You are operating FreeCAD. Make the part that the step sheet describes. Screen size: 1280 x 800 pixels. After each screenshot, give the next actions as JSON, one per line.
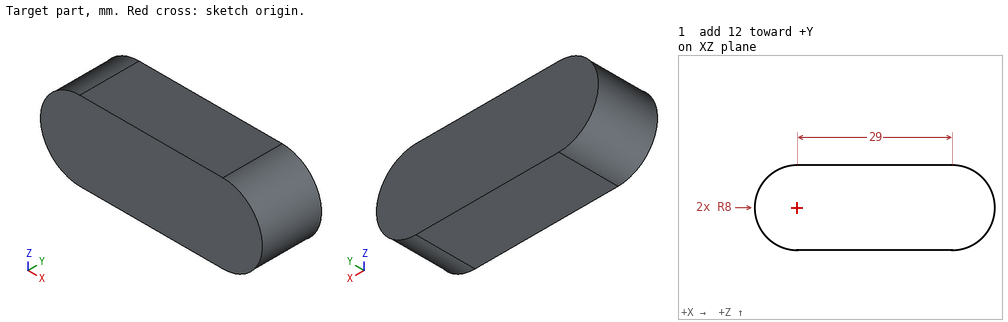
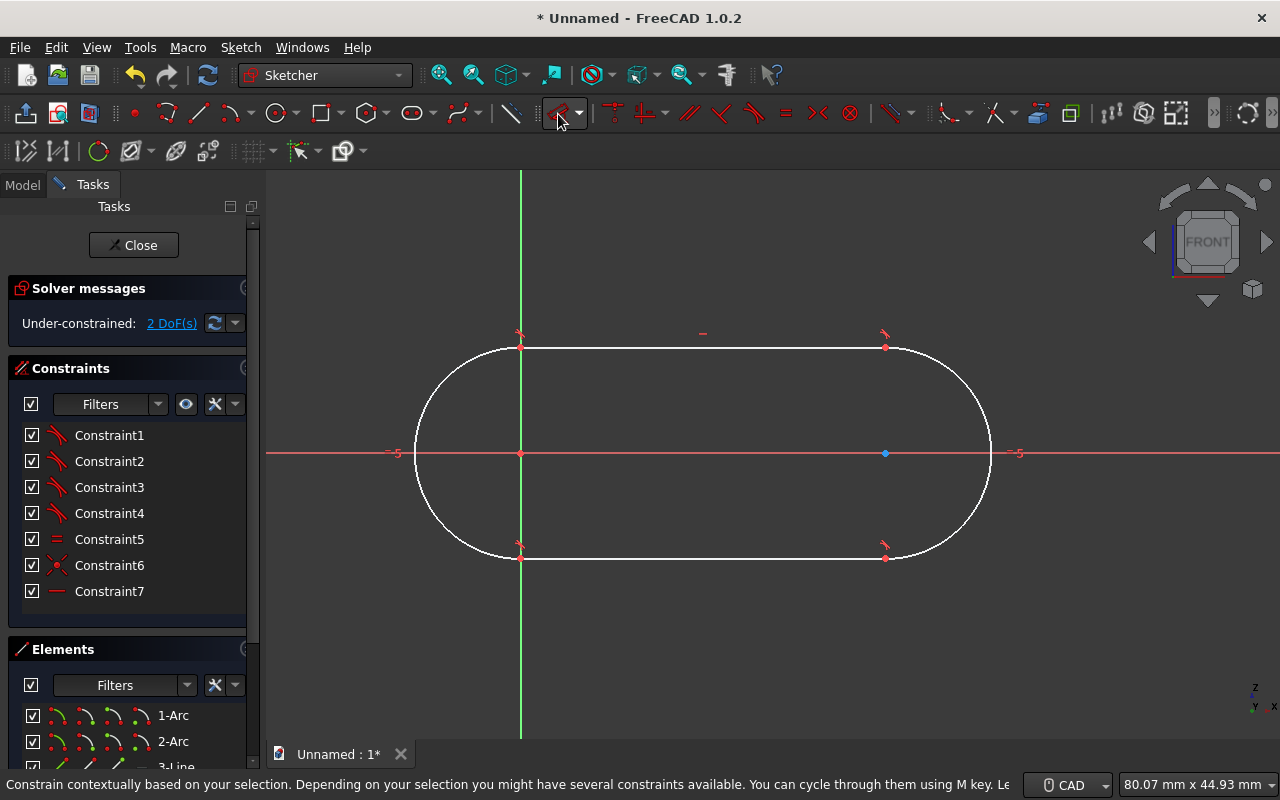
{"action": "left_click", "coordinate": [435, 391]}
{"action": "left_click", "coordinate": [409, 372]}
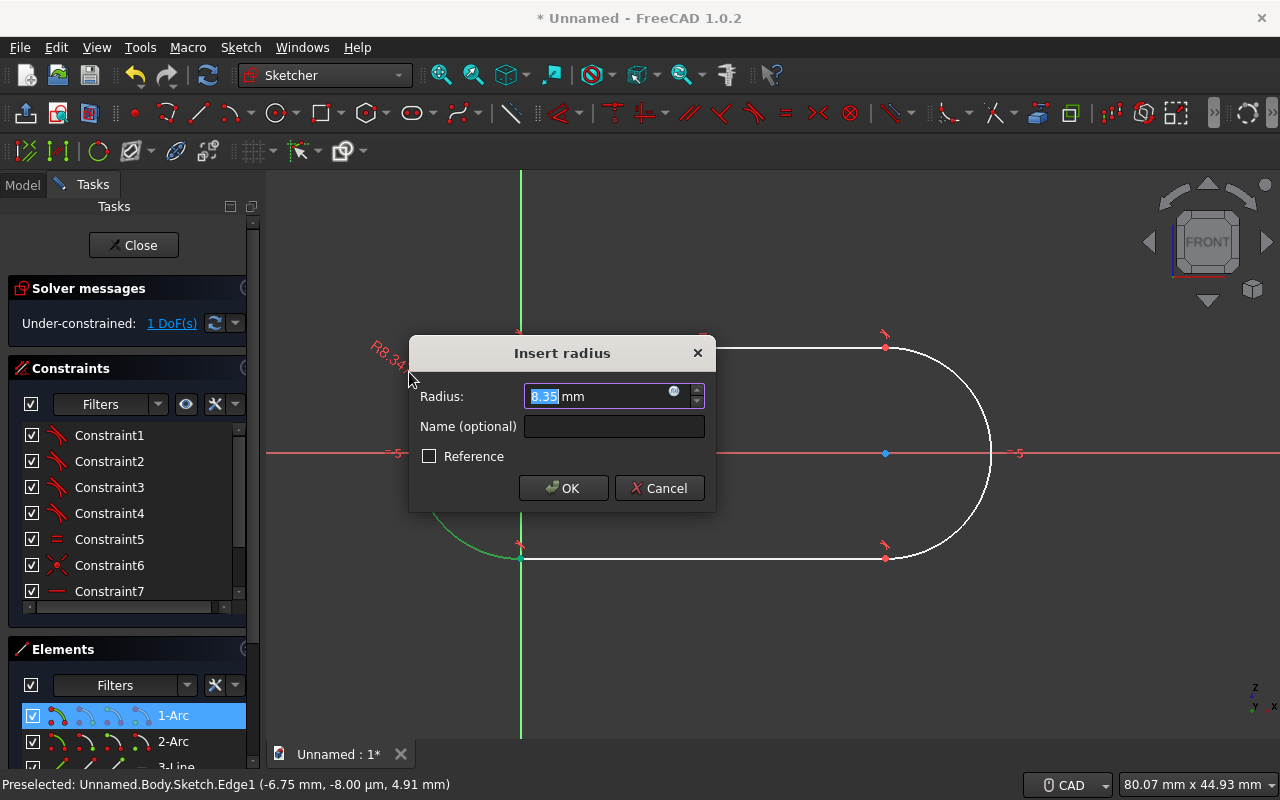
{"action": "type", "text": "8"}
{"action": "key", "text": "Return"}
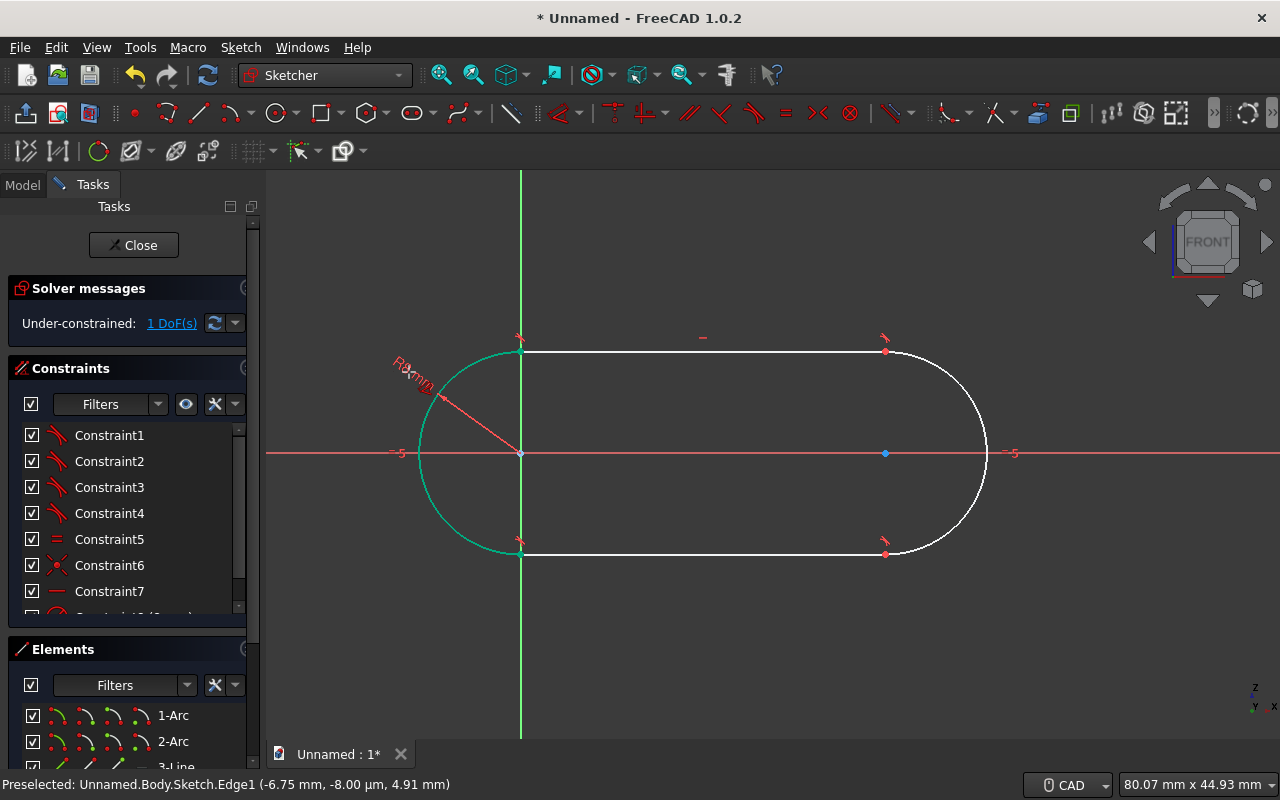
{"action": "left_click", "coordinate": [630, 352]}
{"action": "left_click", "coordinate": [703, 318]}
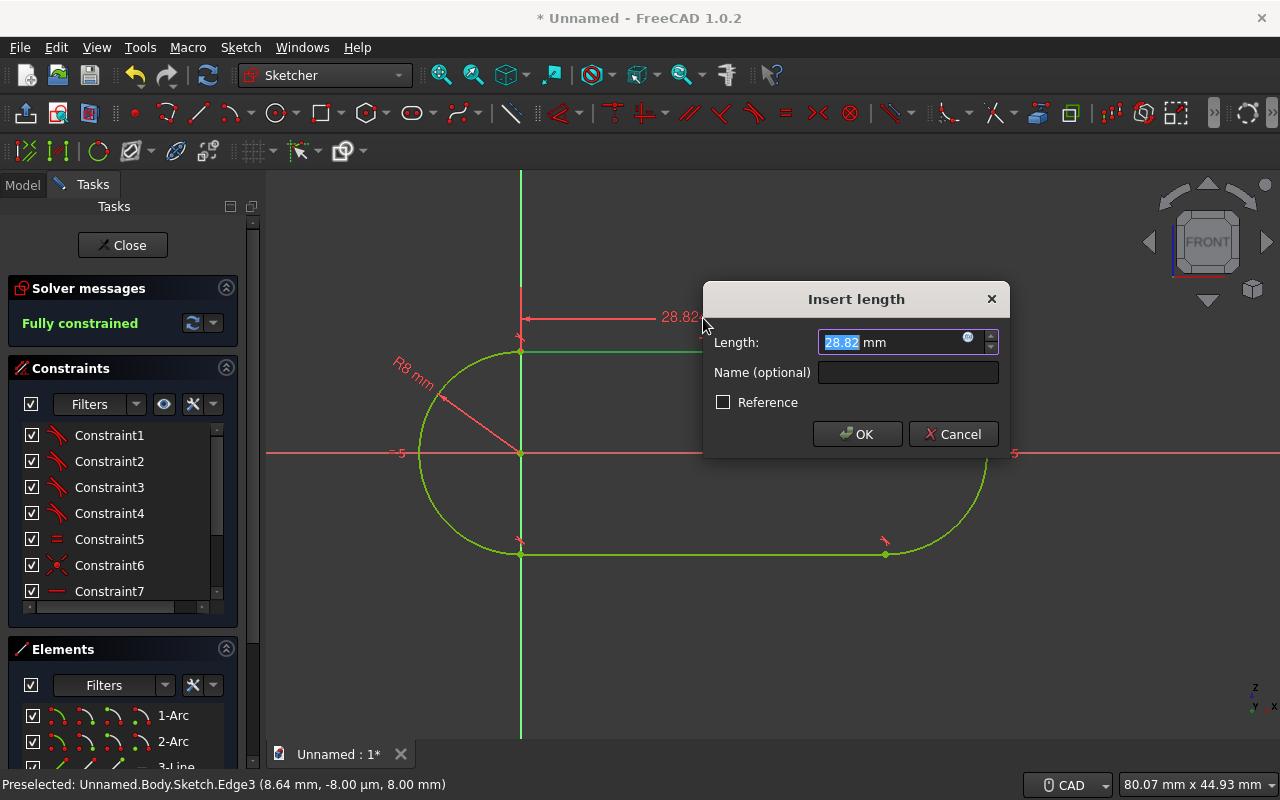
{"action": "type", "text": "29"}
{"action": "key", "text": "Return"}
{"action": "key", "text": "Escape"}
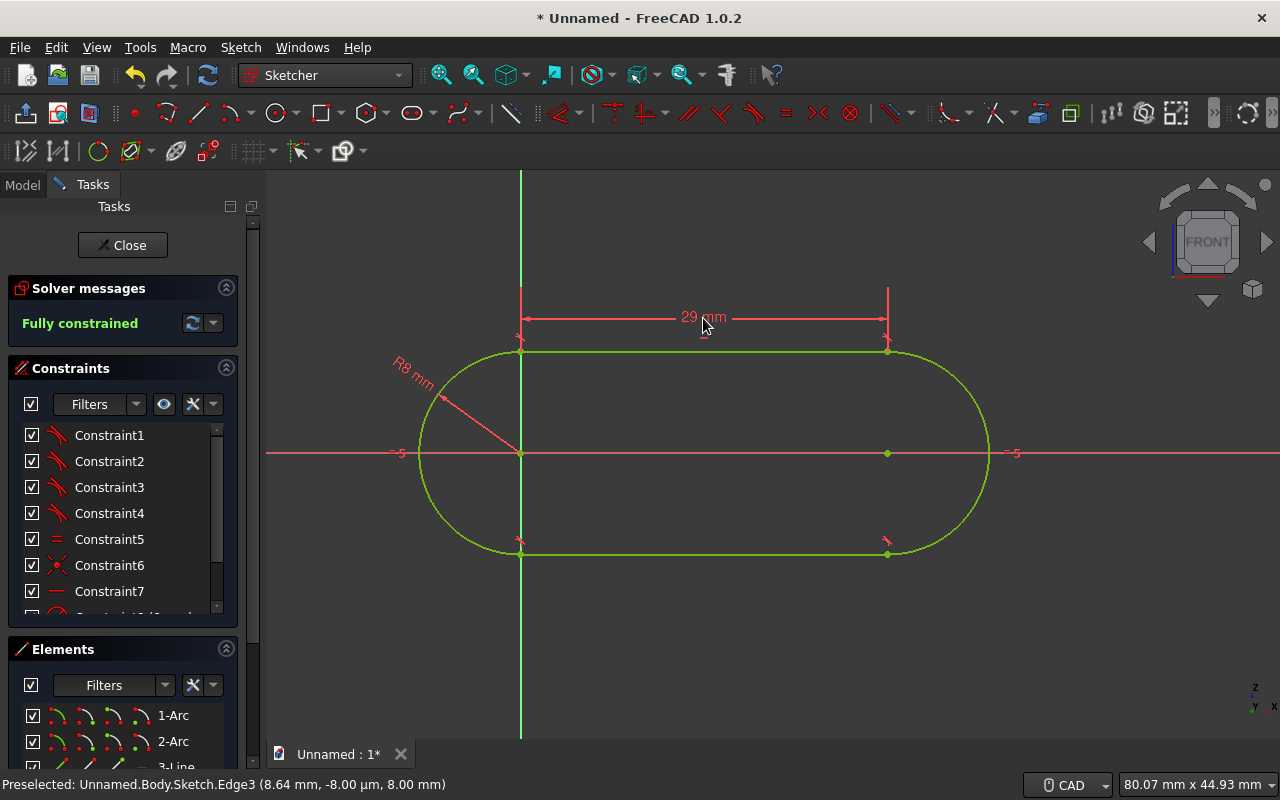
{"action": "left_click", "coordinate": [123, 245]}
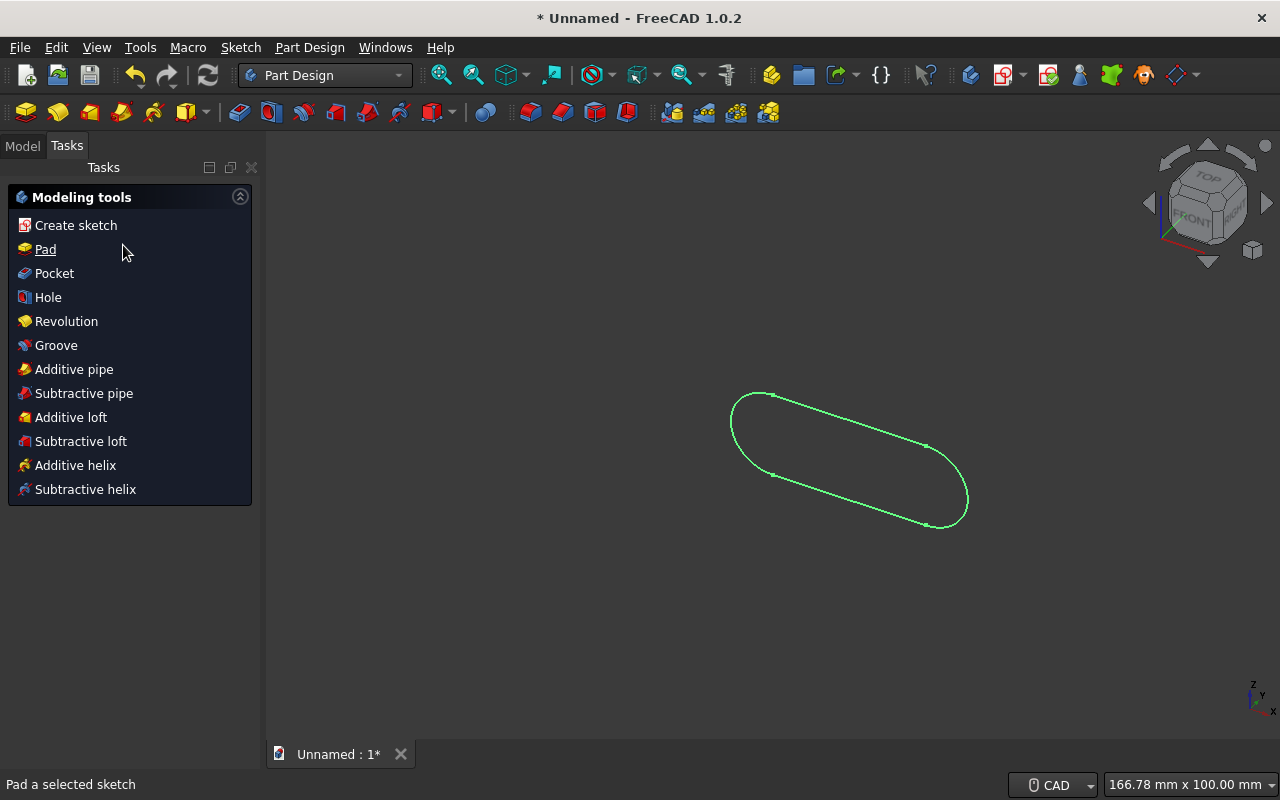
{"action": "left_click", "coordinate": [26, 112]}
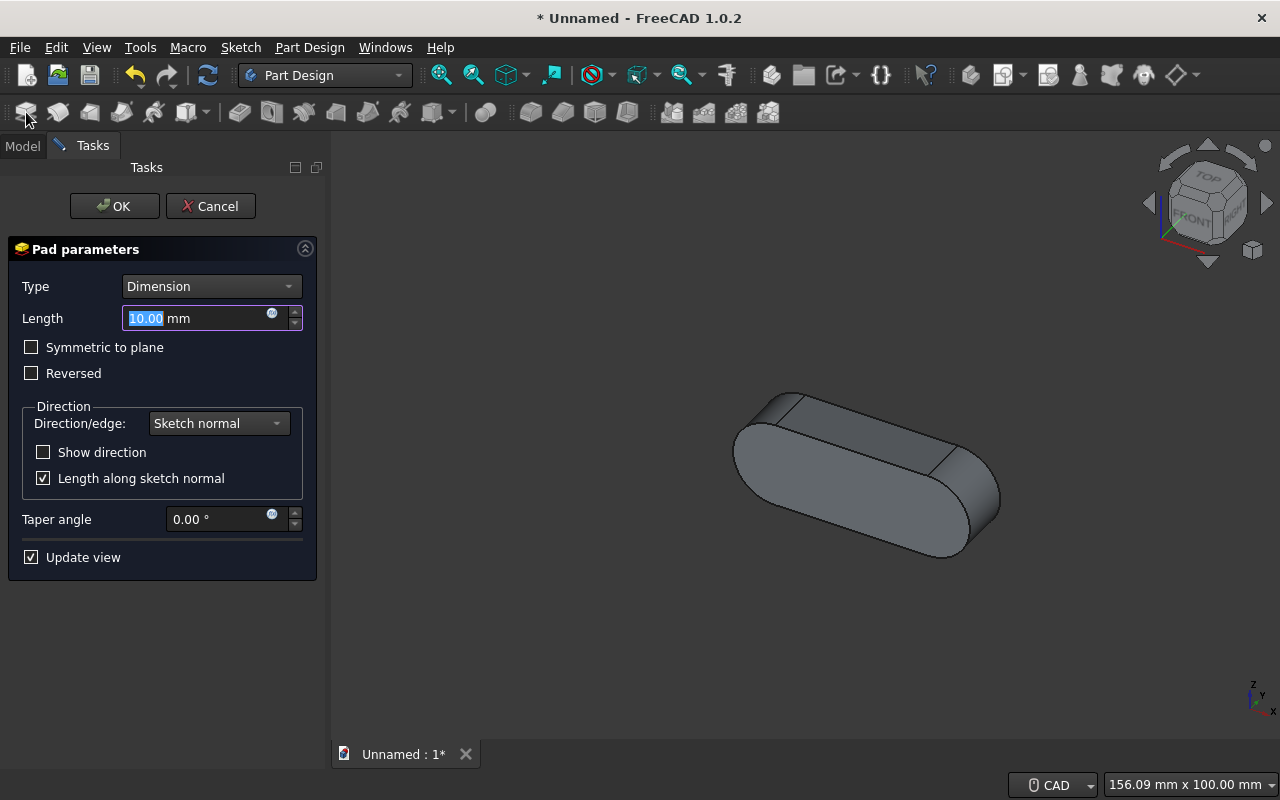
{"action": "type", "text": "12"}
{"action": "key", "text": "Tab"}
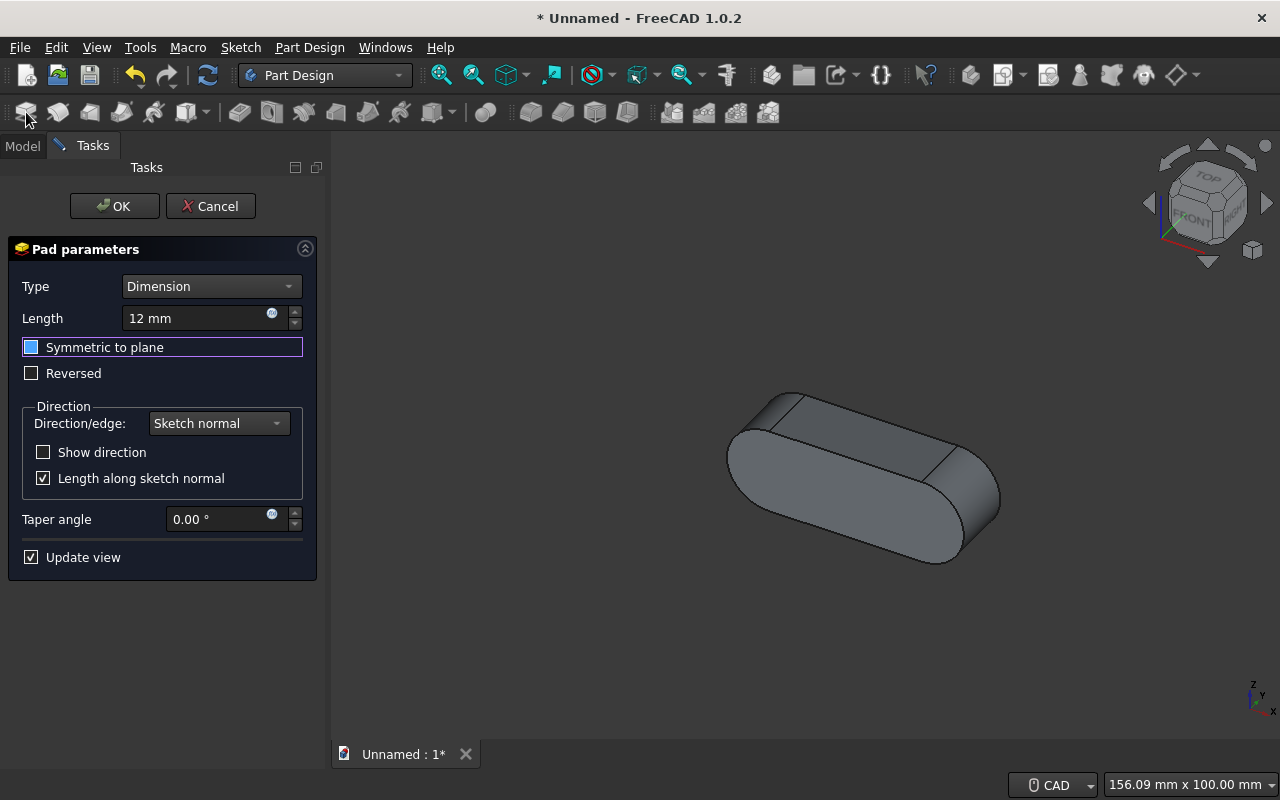
{"action": "left_click", "coordinate": [30, 373]}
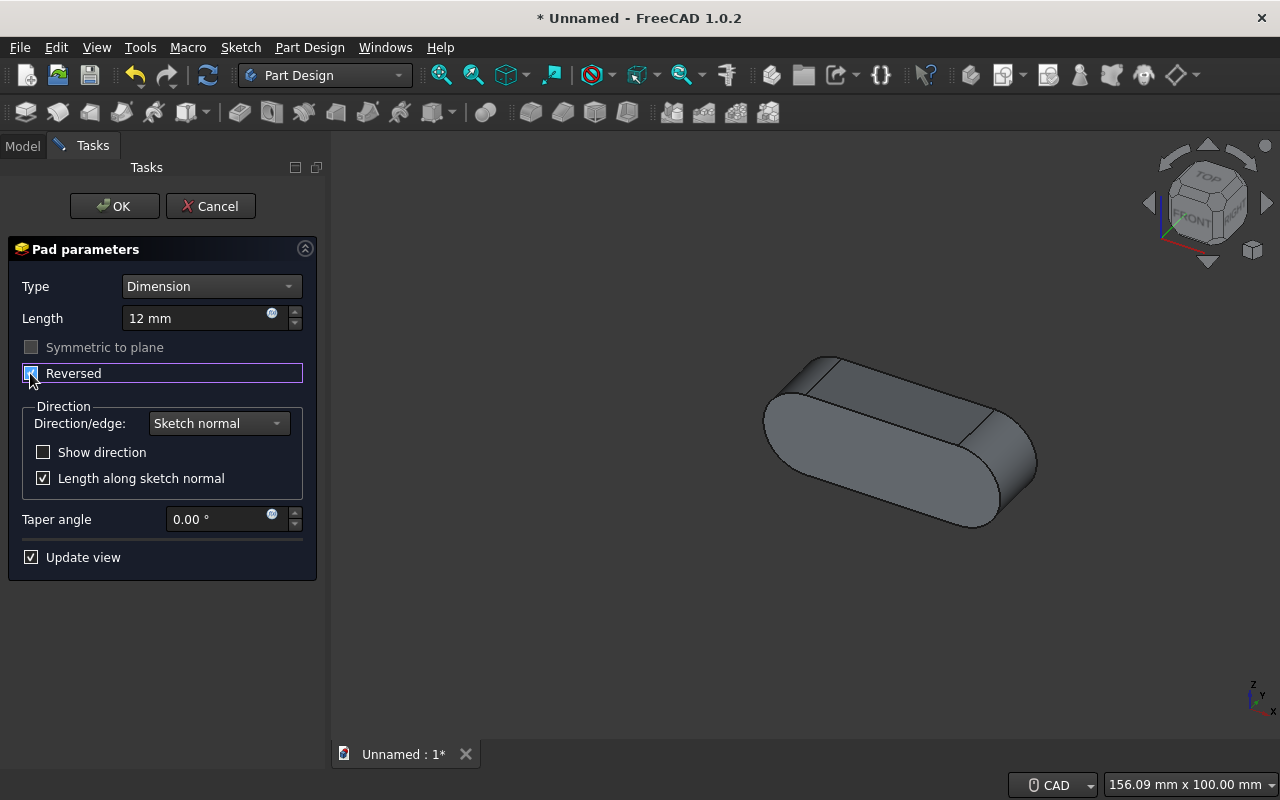
{"action": "left_click", "coordinate": [115, 206]}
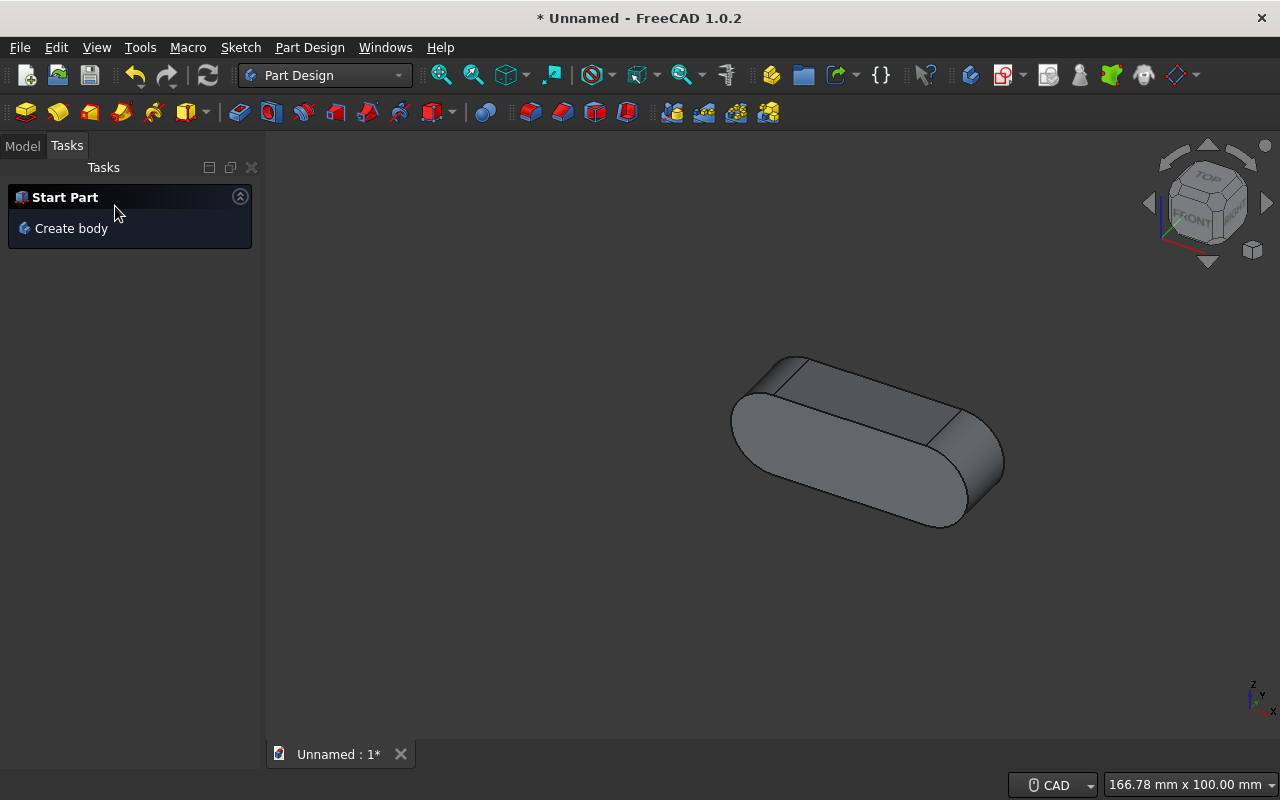
{"action": "key", "text": "0"}